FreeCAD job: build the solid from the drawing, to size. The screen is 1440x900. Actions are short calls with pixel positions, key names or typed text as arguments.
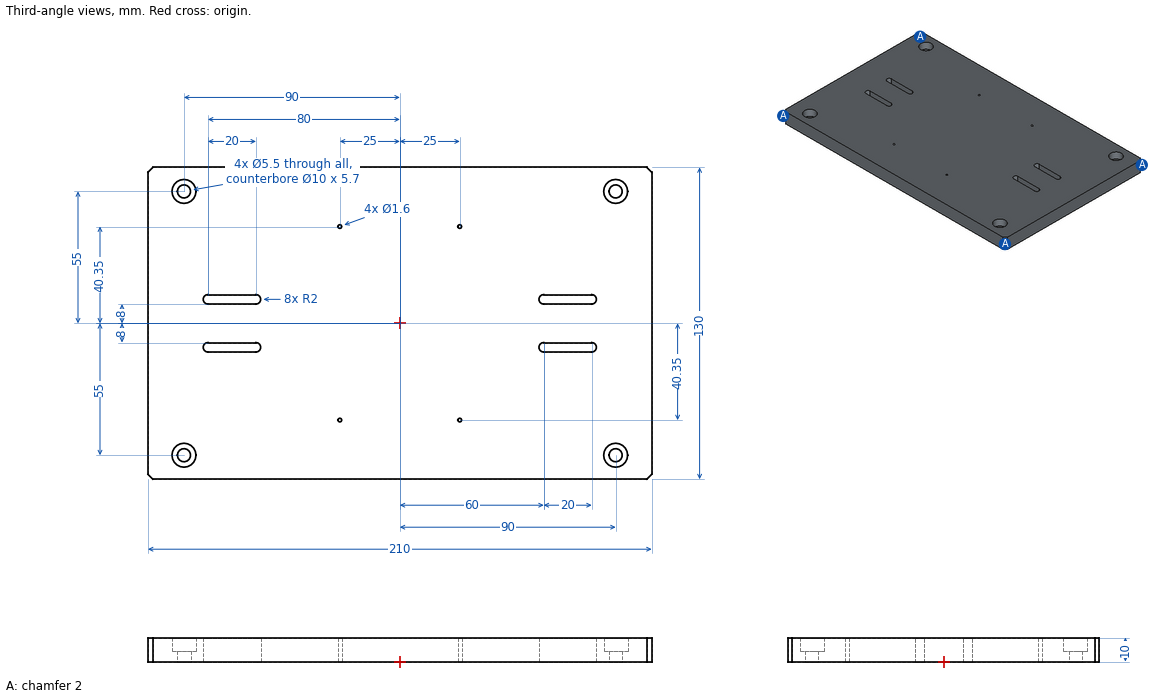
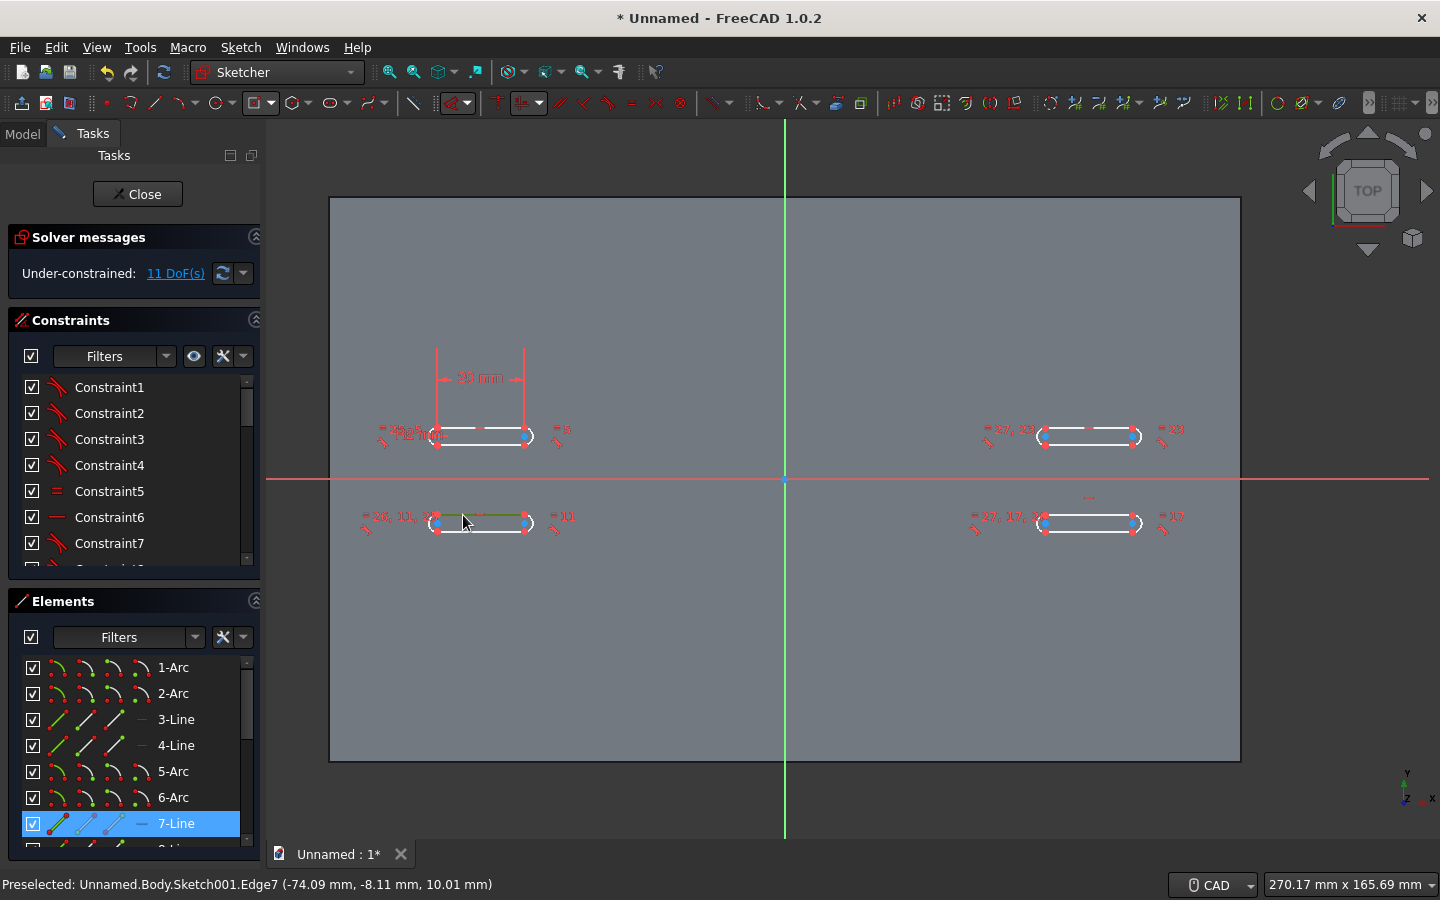
click(470, 104)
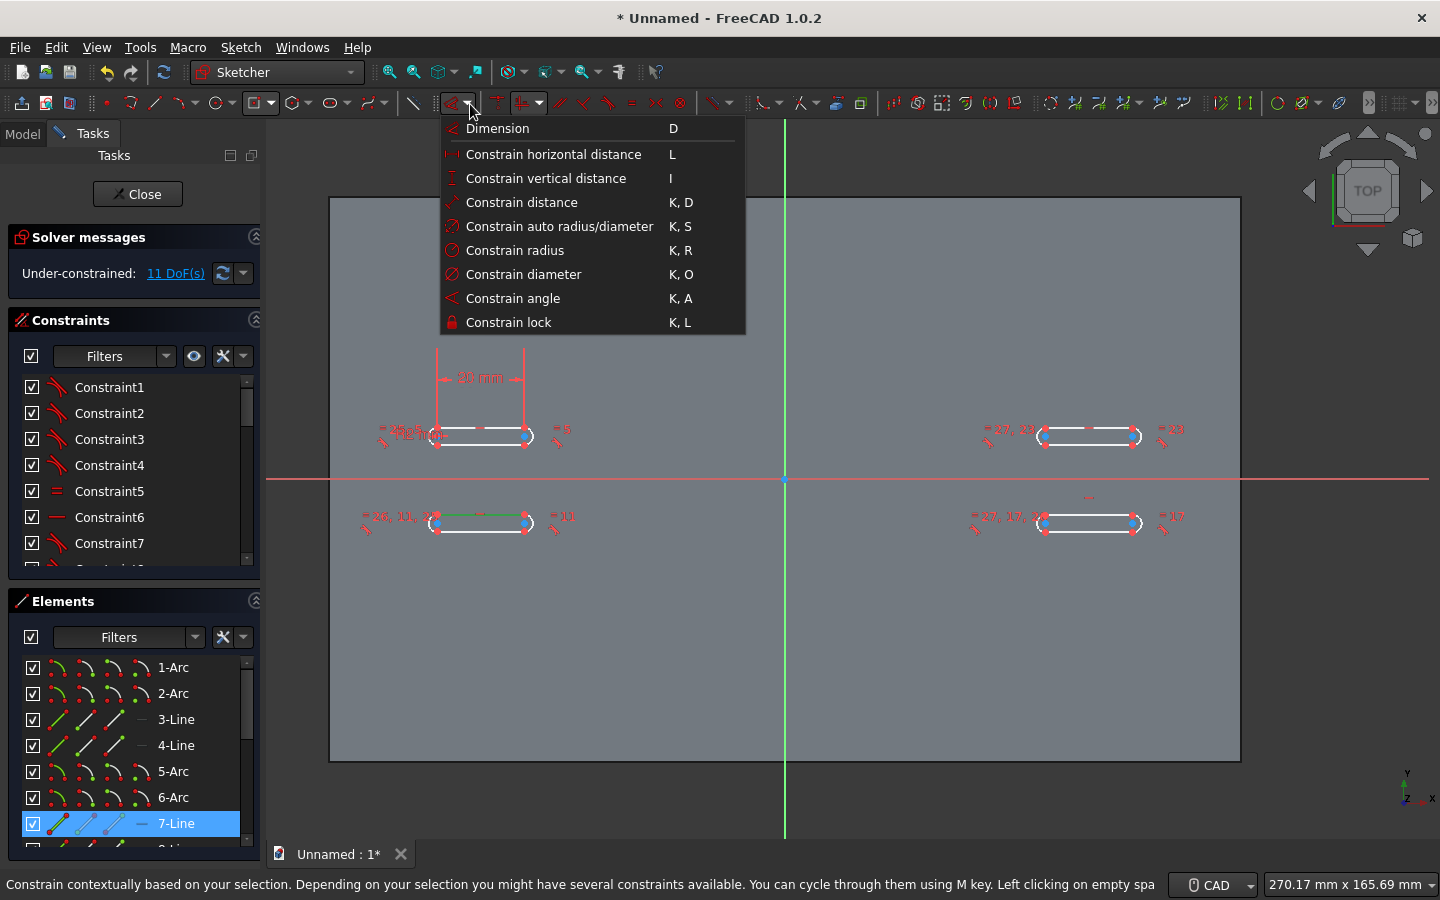
click(593, 154)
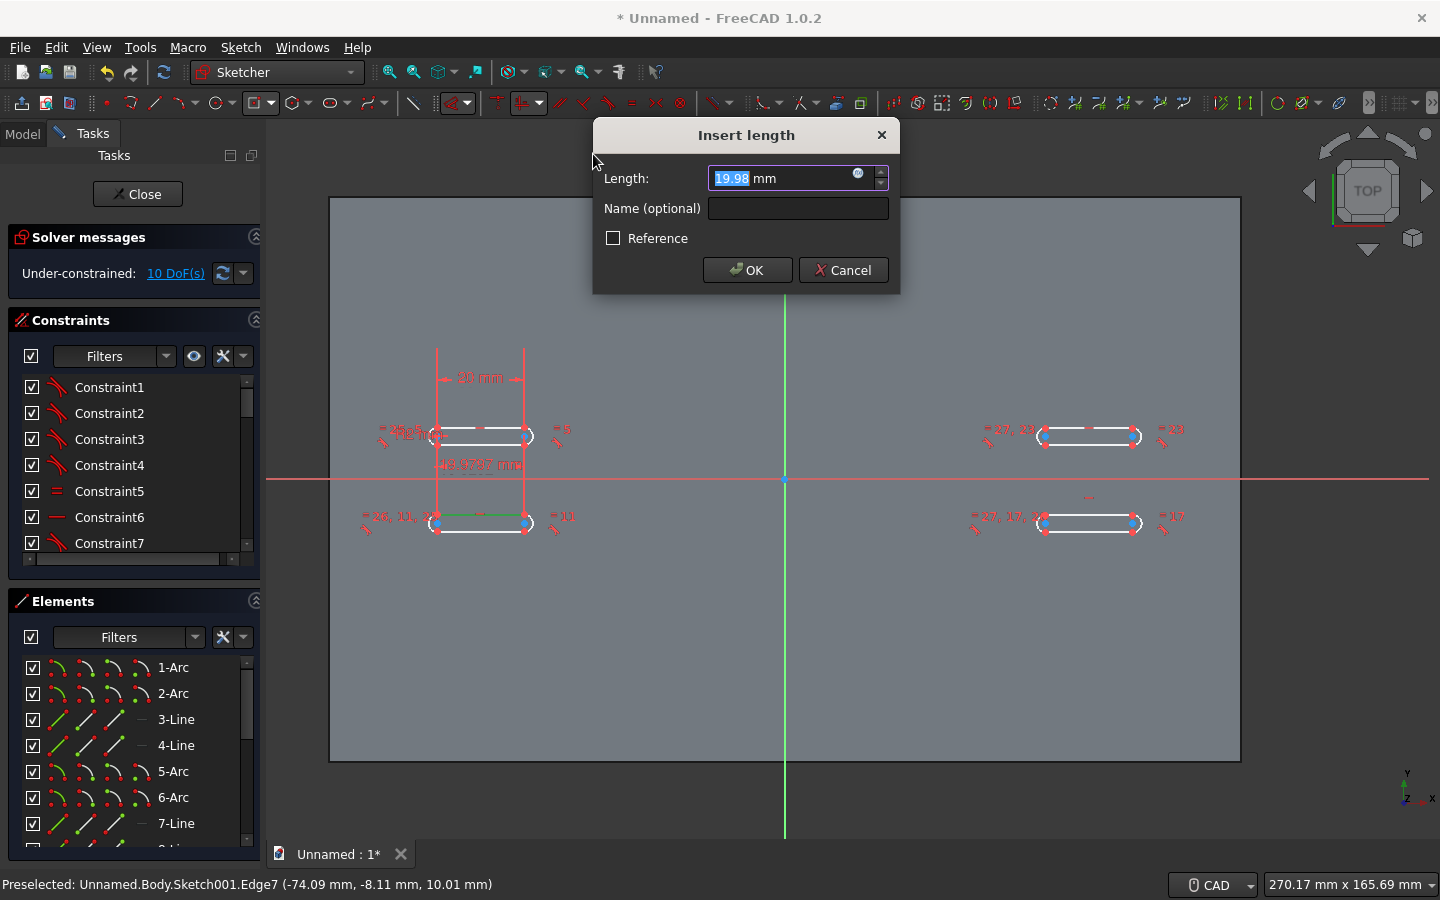
text(20)
key(Return)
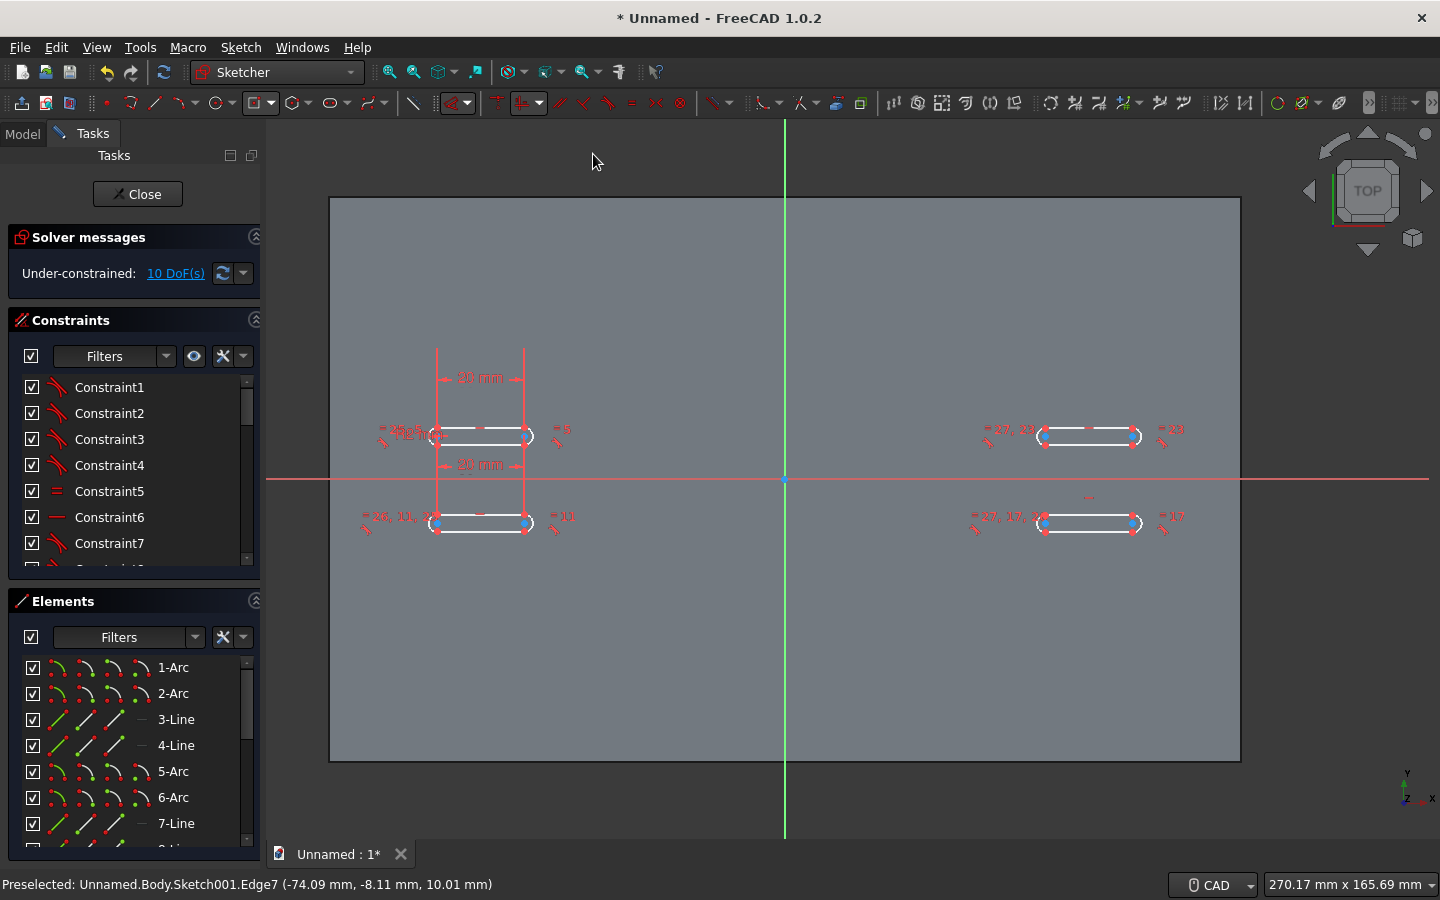
click(1072, 515)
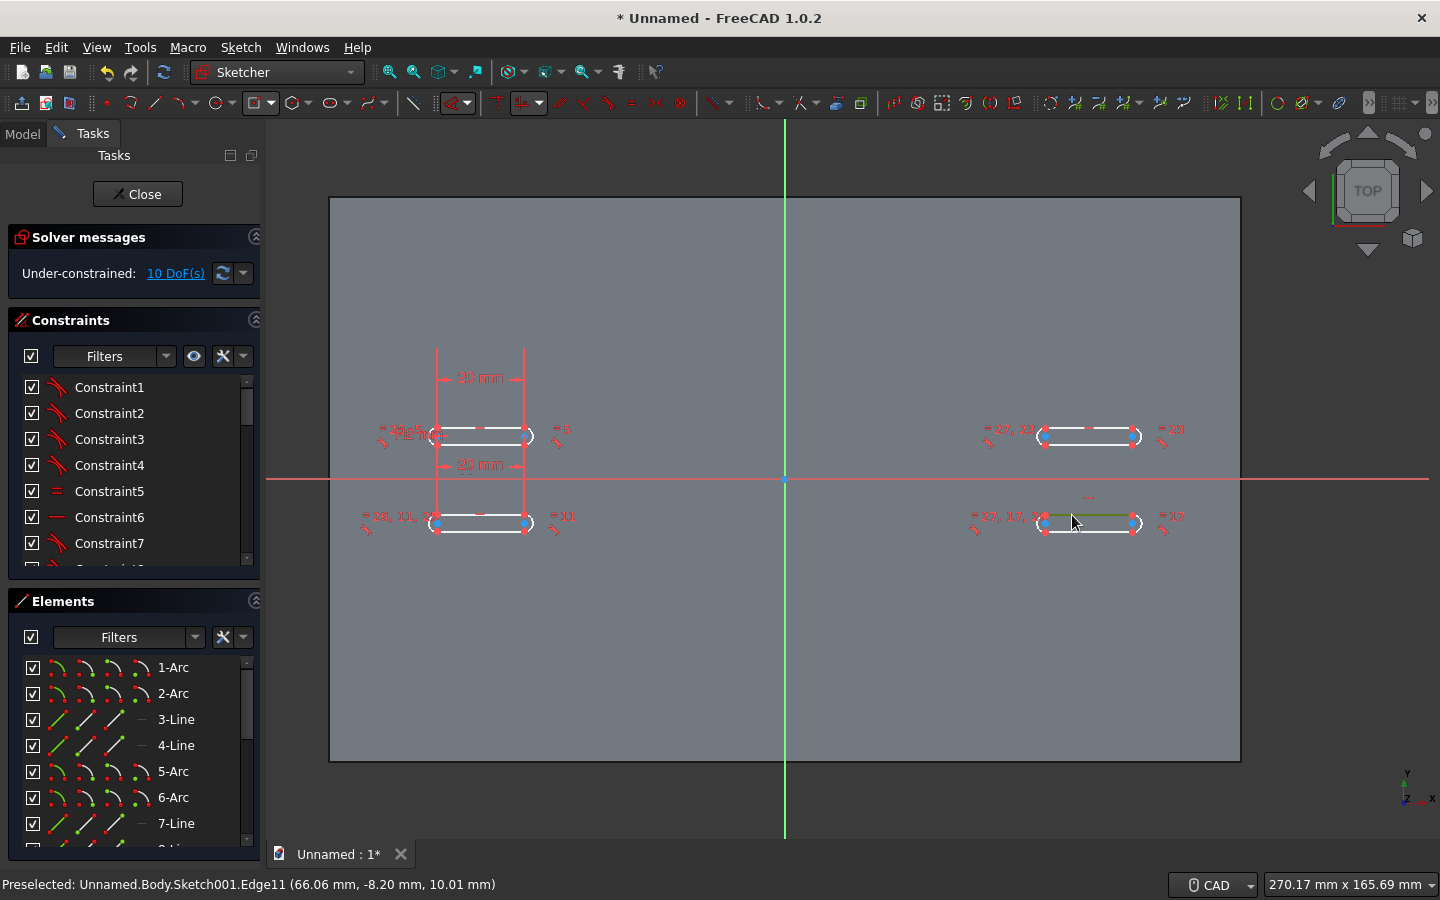
click(470, 104)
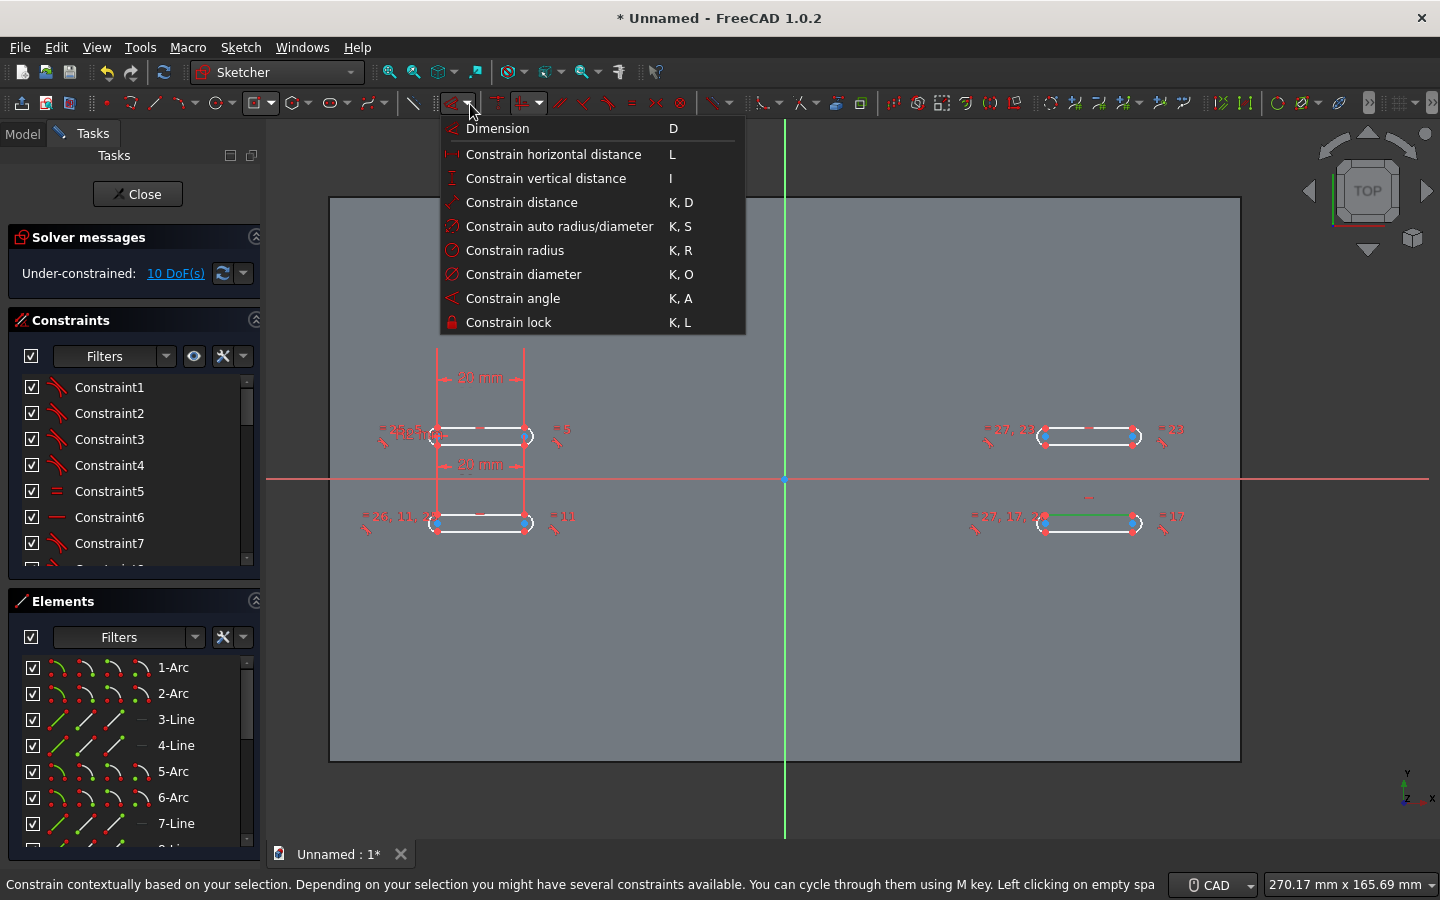
click(593, 154)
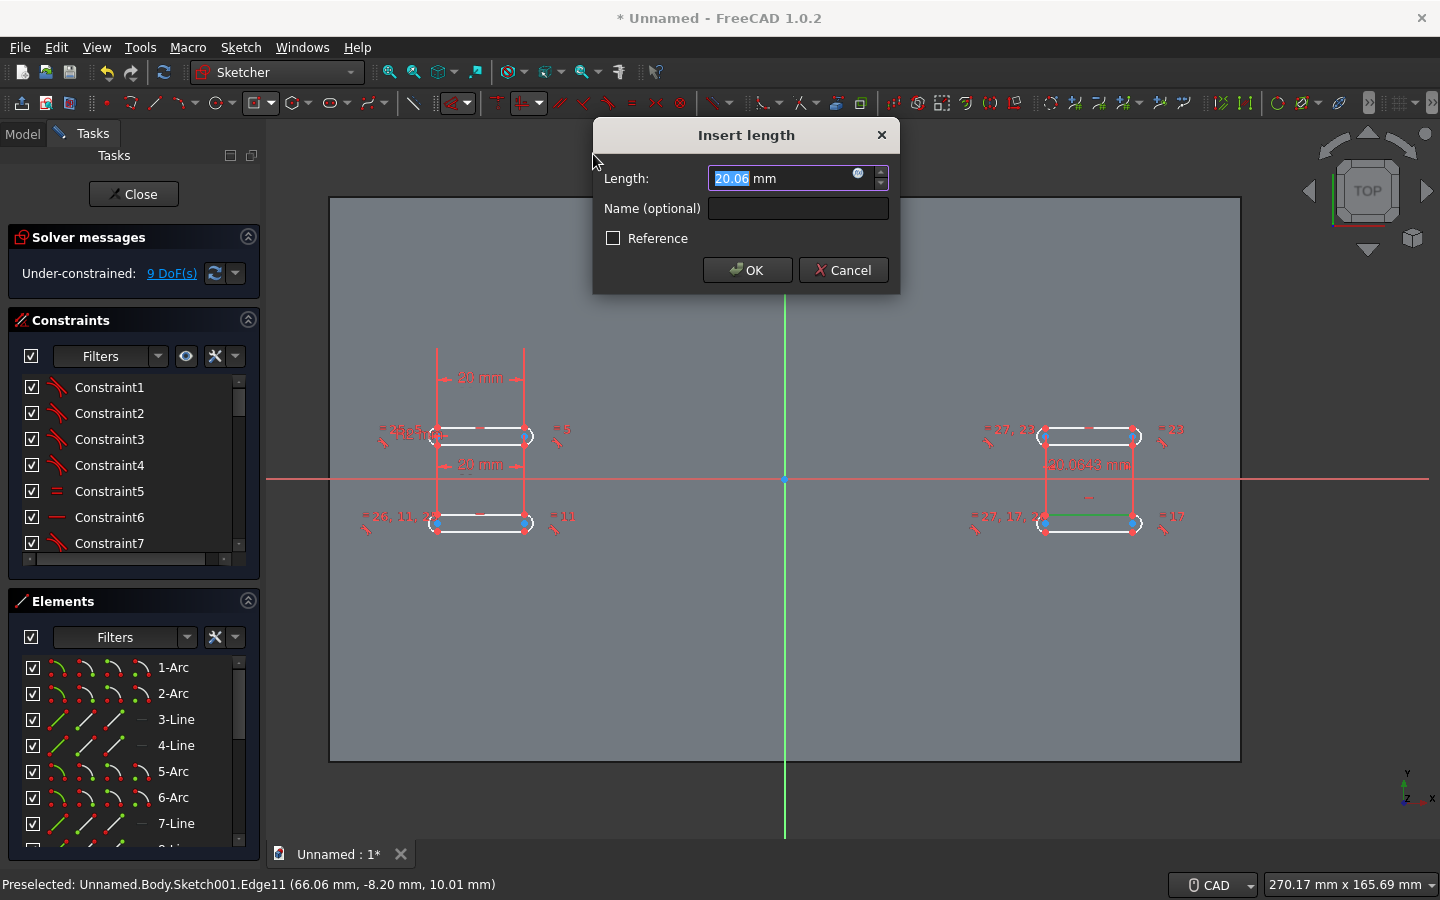
text(20)
key(Return)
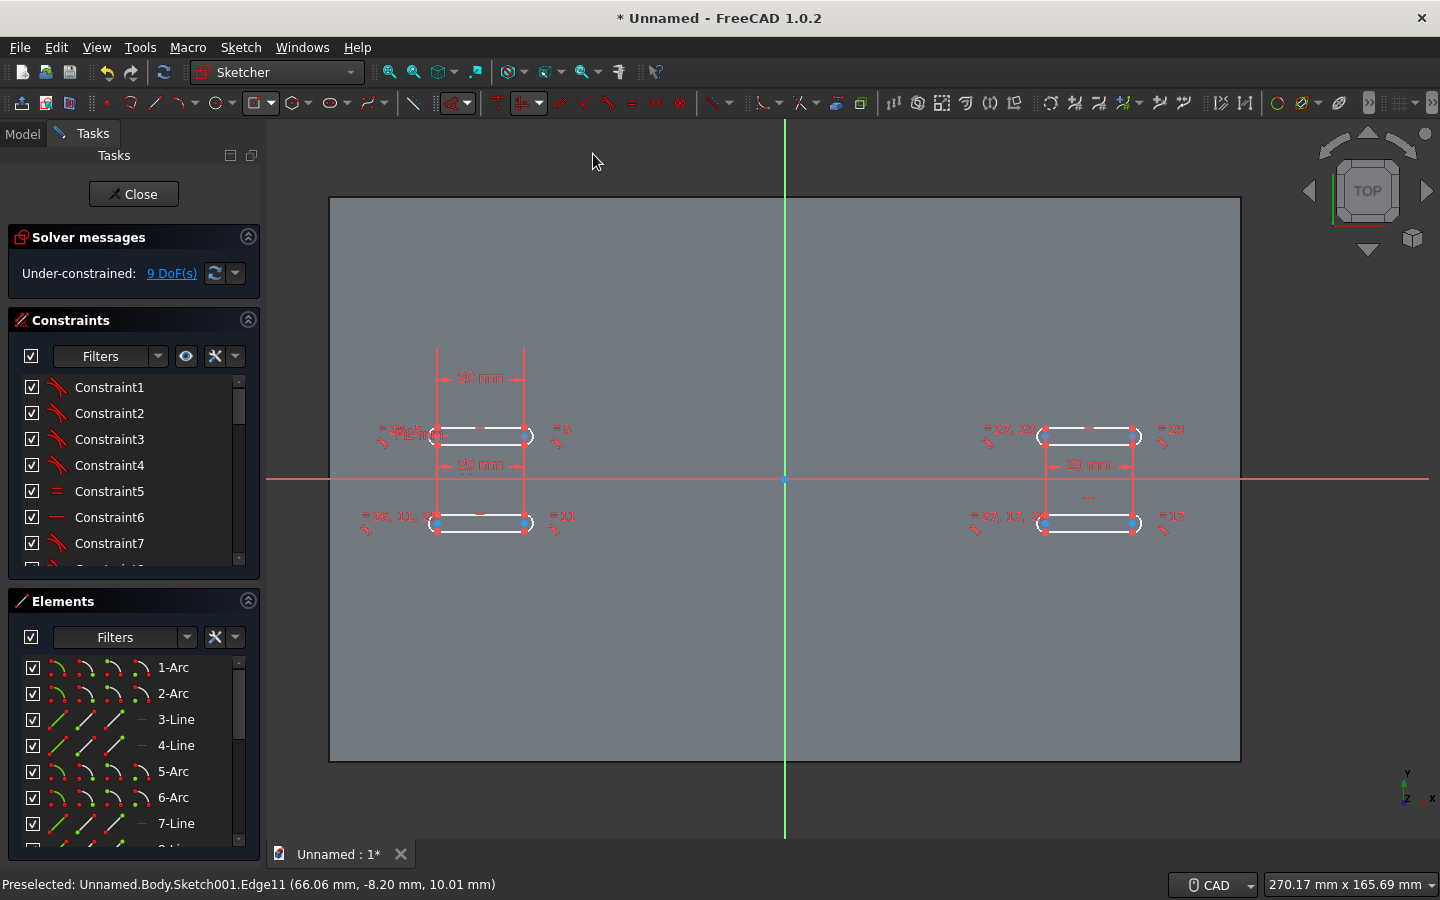
click(1072, 428)